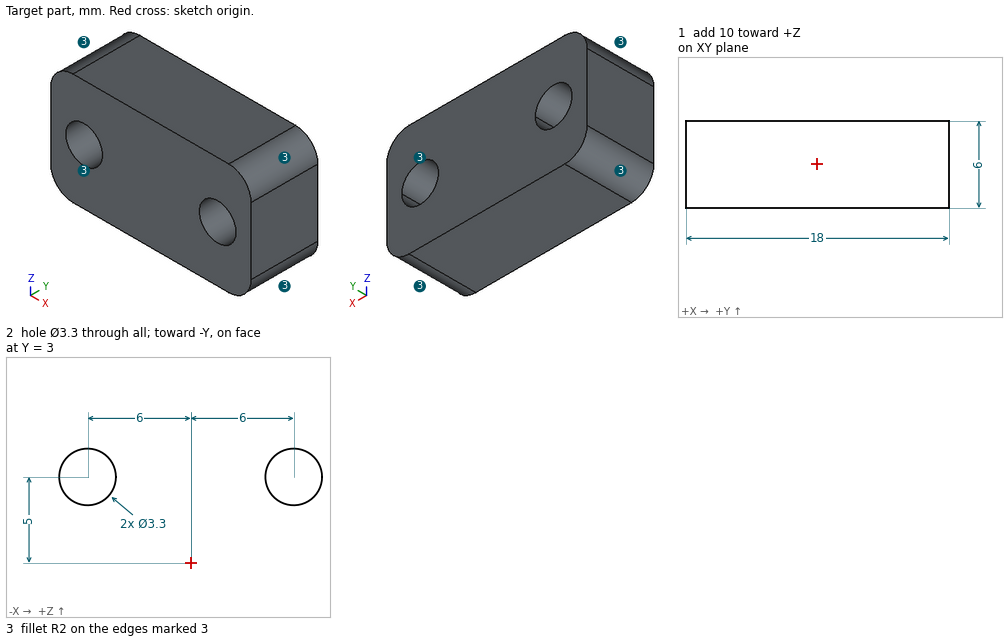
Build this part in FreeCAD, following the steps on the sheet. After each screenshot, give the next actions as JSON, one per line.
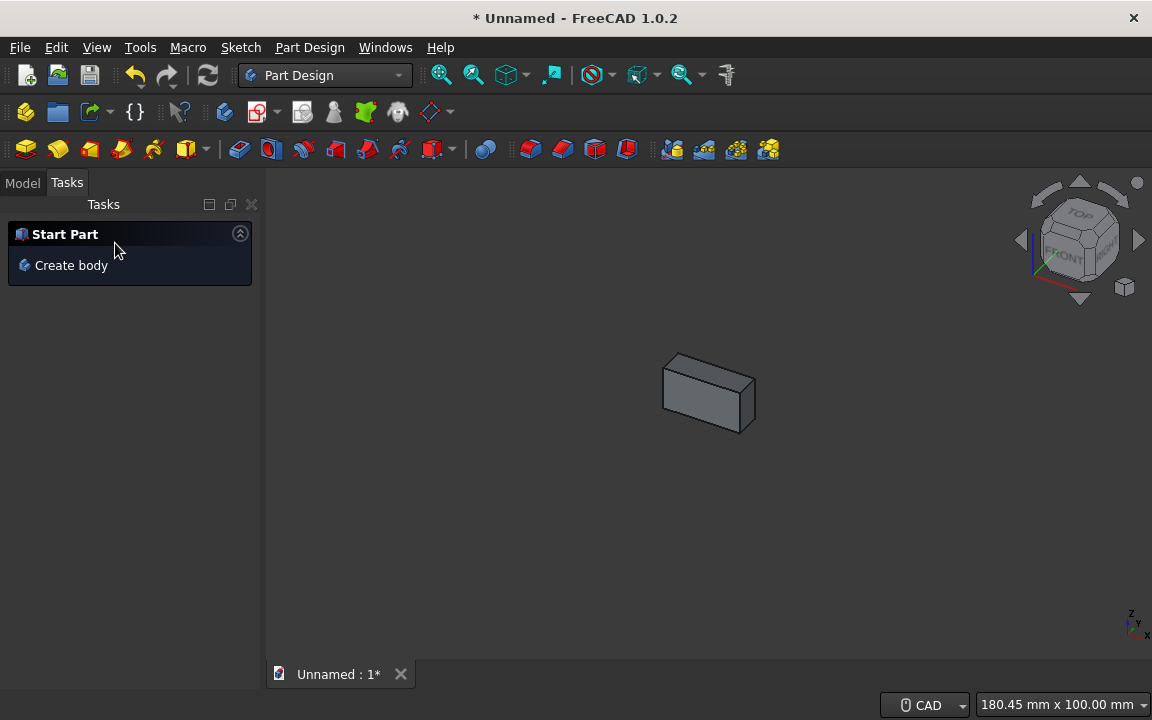
{"action": "key", "text": "v f"}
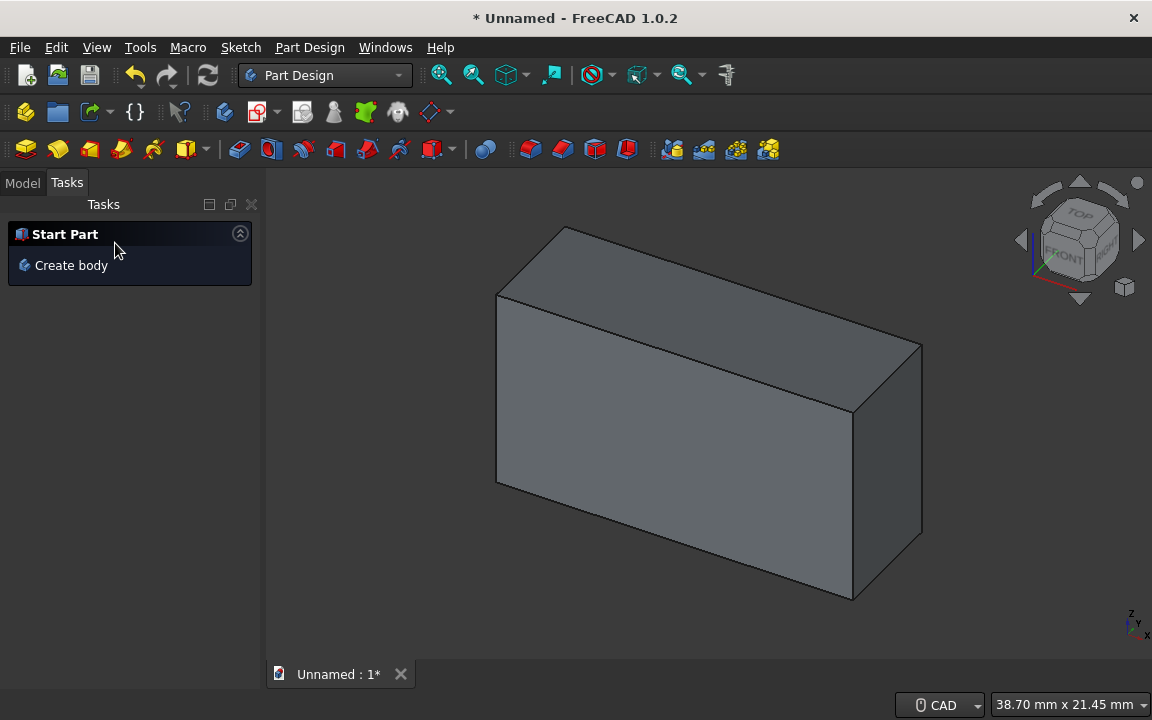
{"action": "key", "text": "4"}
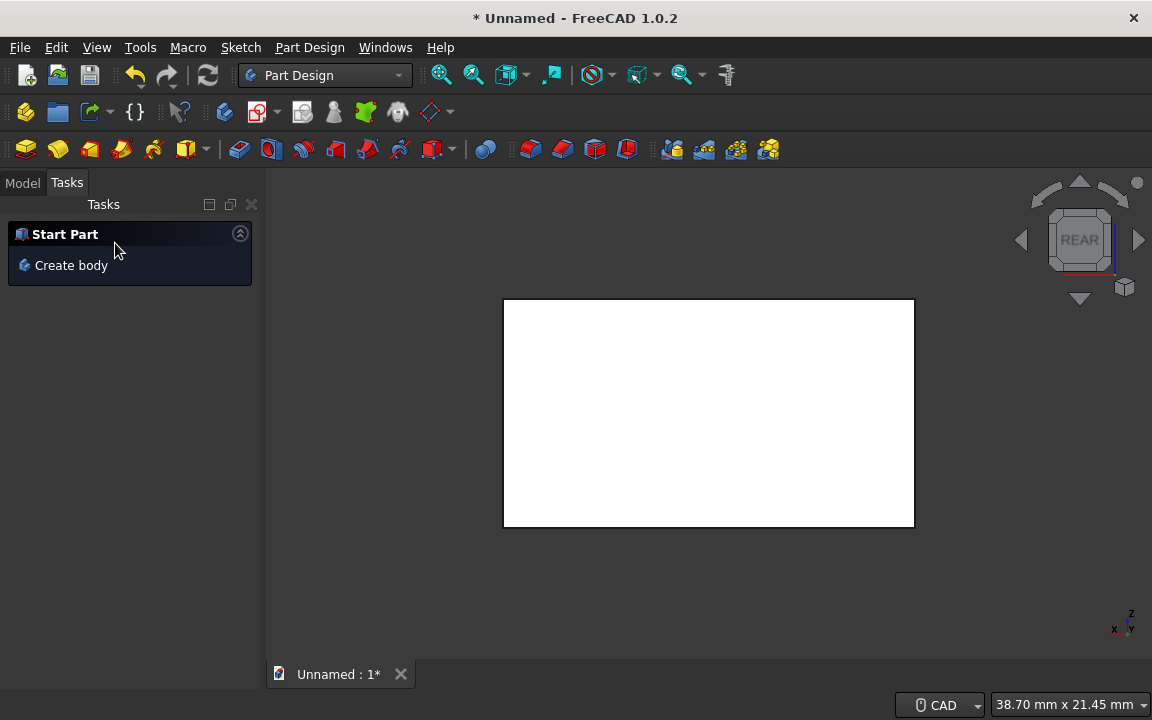
{"action": "left_click", "coordinate": [650, 413]}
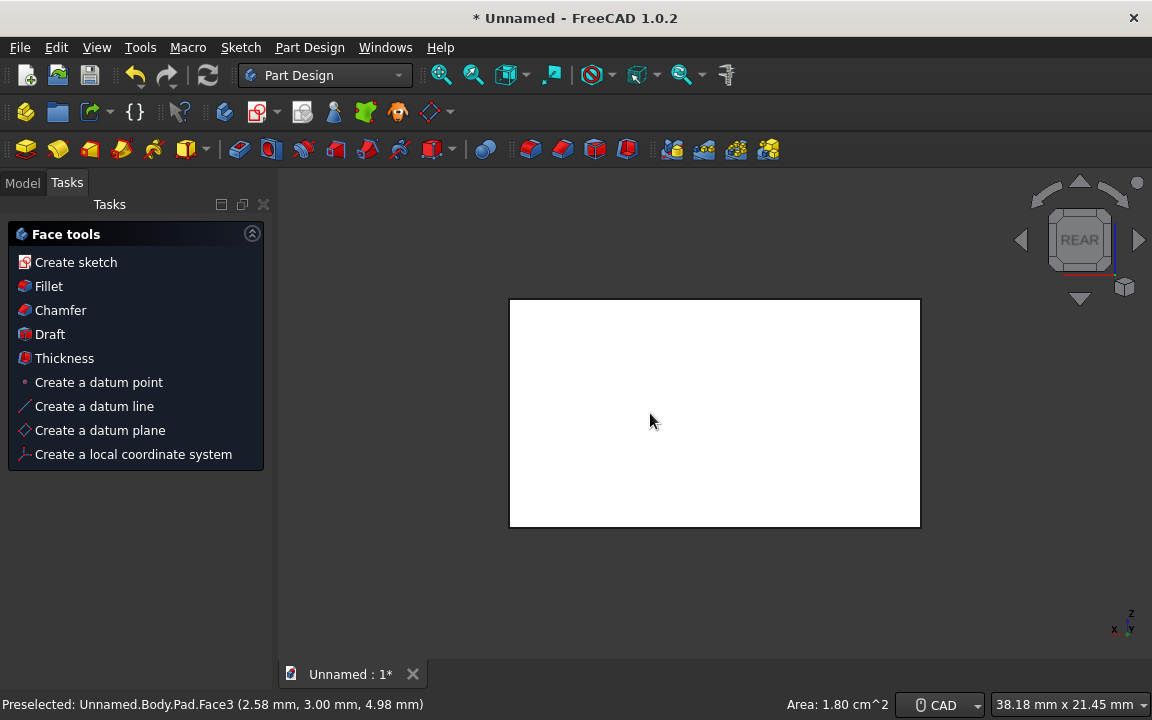
{"action": "left_click", "coordinate": [258, 112]}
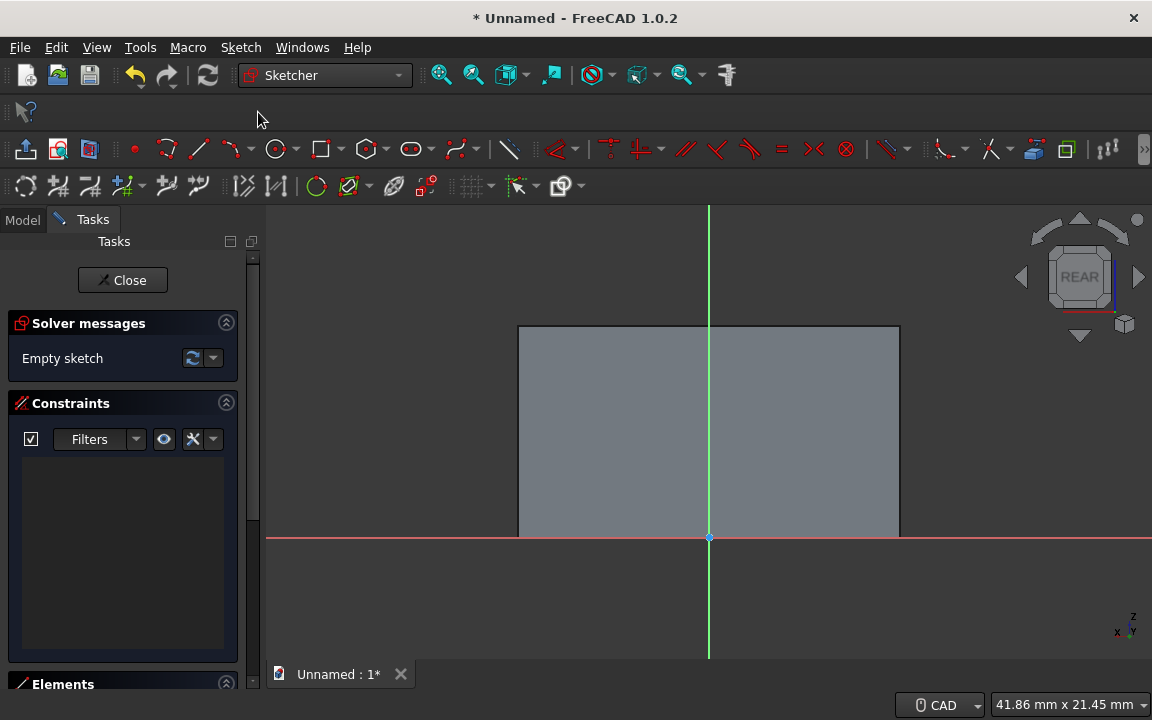
{"action": "scroll", "coordinate": [848, 540], "scroll_direction": "up", "scroll_amount": 2}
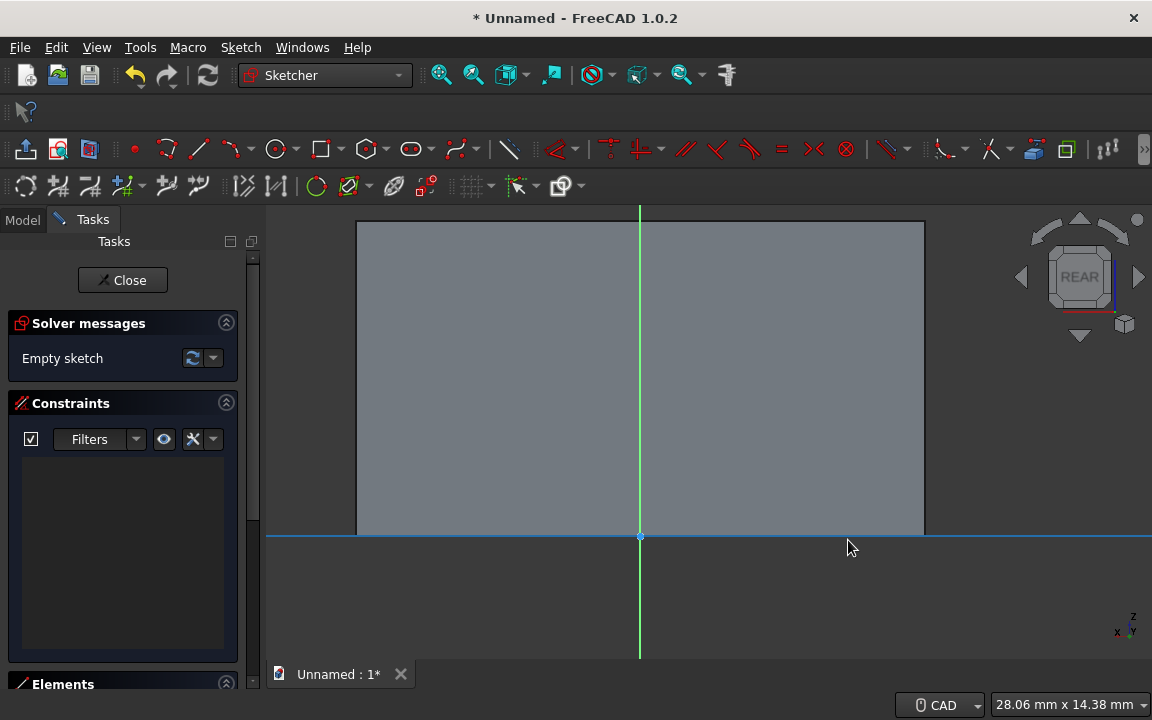
{"action": "left_click", "coordinate": [276, 150]}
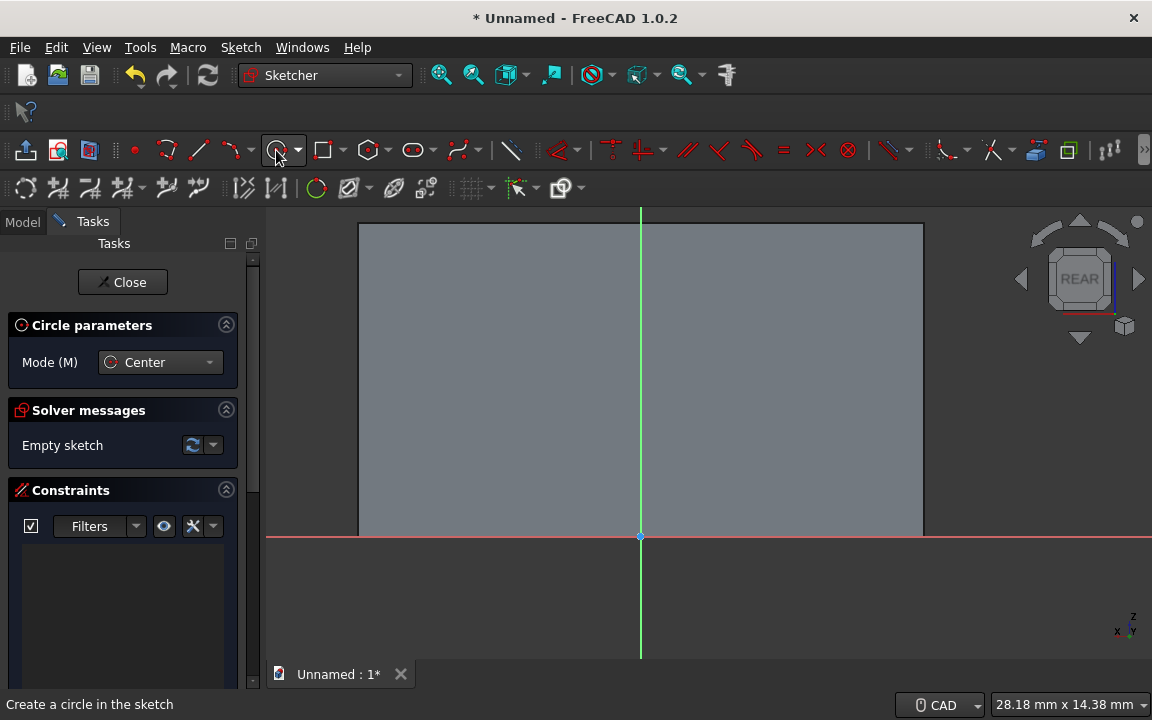
{"action": "left_click", "coordinate": [452, 380]}
{"action": "mouse_move", "coordinate": [489, 343]}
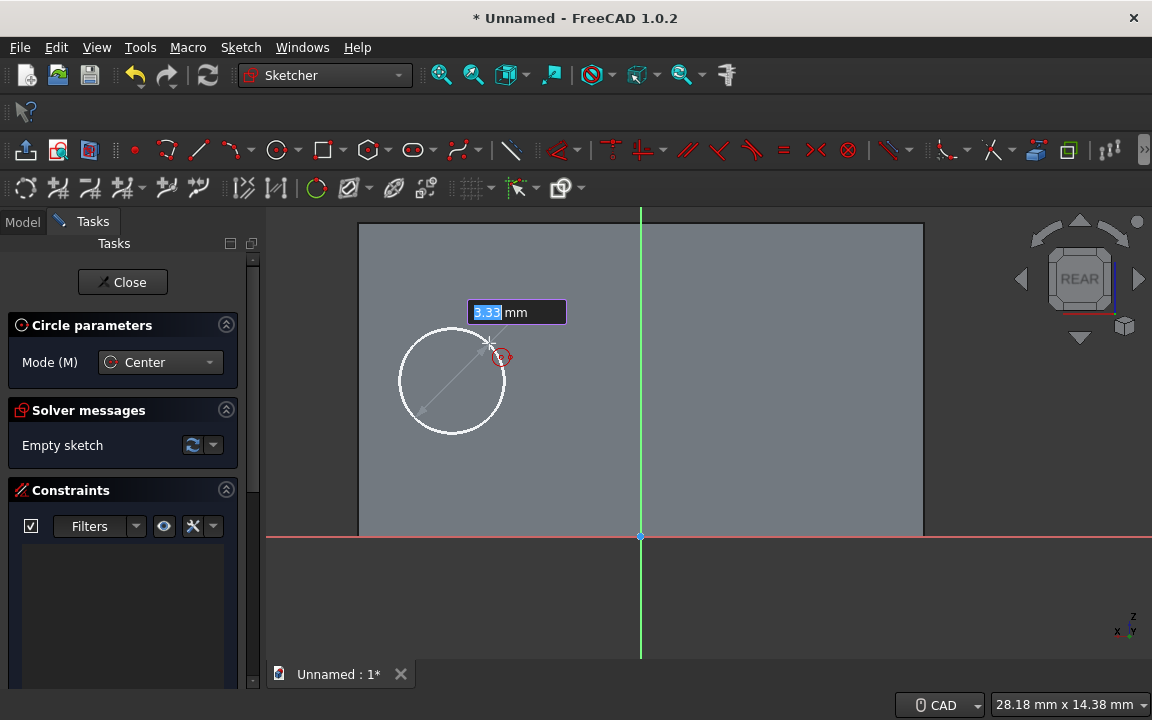
{"action": "type", "text": "3.3"}
{"action": "key", "text": "Return"}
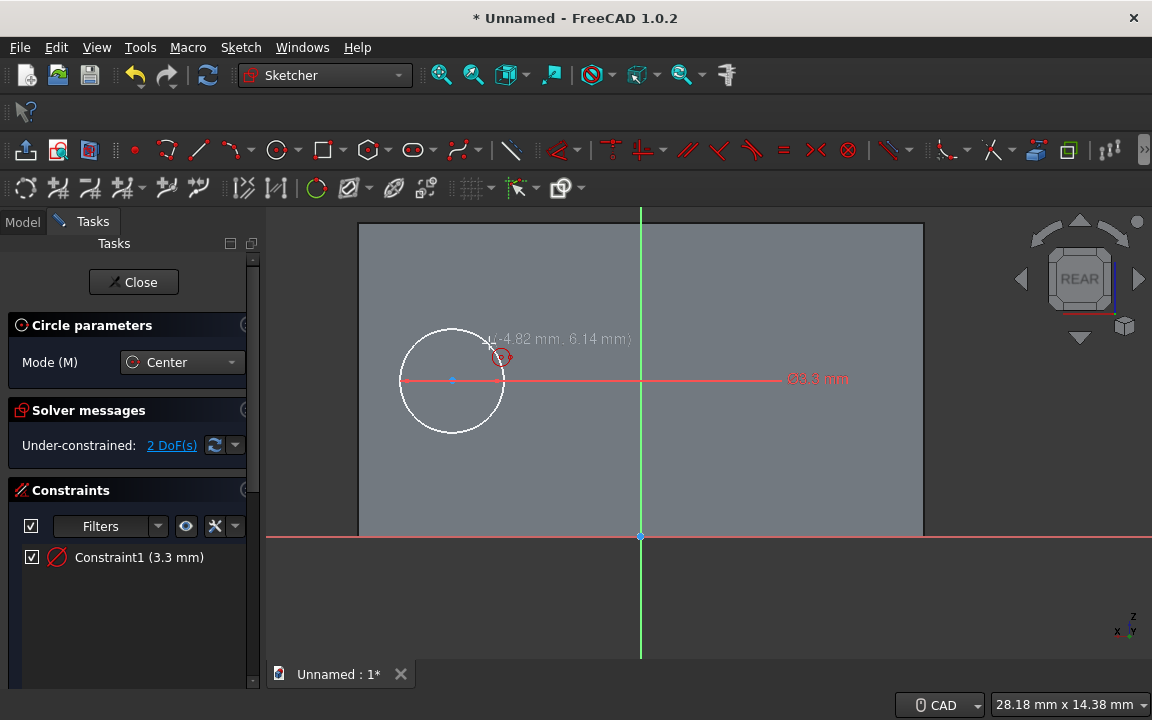
{"action": "left_click", "coordinate": [829, 380]}
{"action": "mouse_move", "coordinate": [866, 343]}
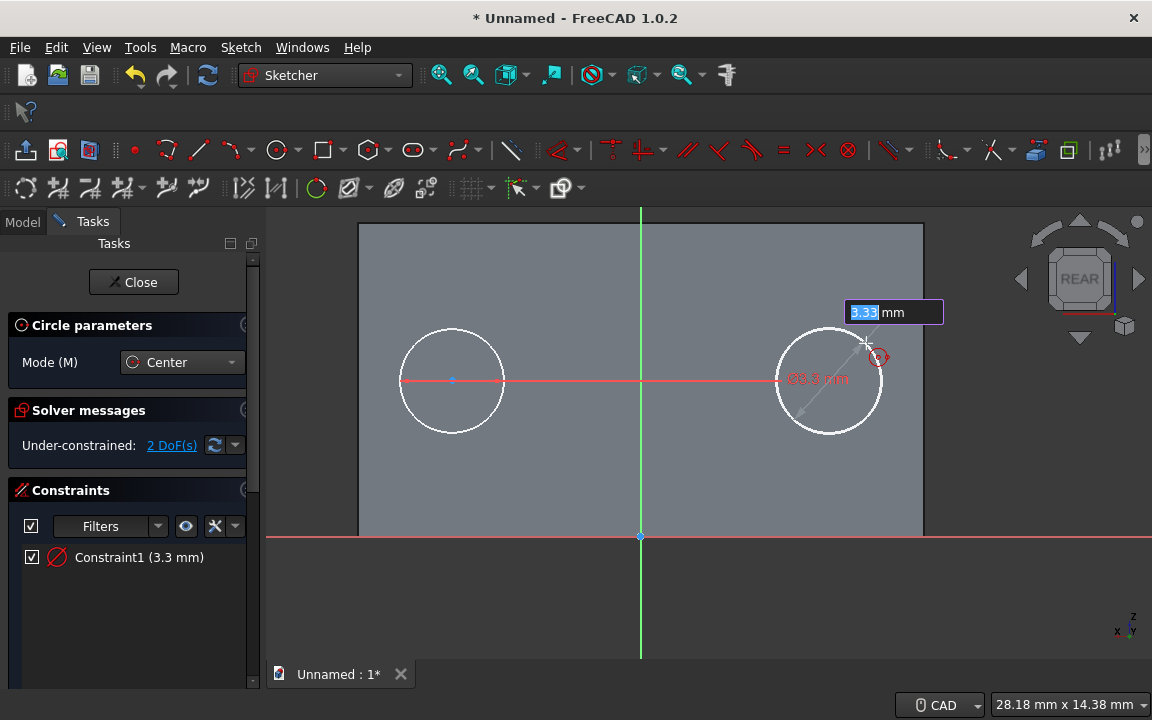
{"action": "type", "text": "3.3"}
{"action": "key", "text": "Return"}
{"action": "key", "text": "Escape"}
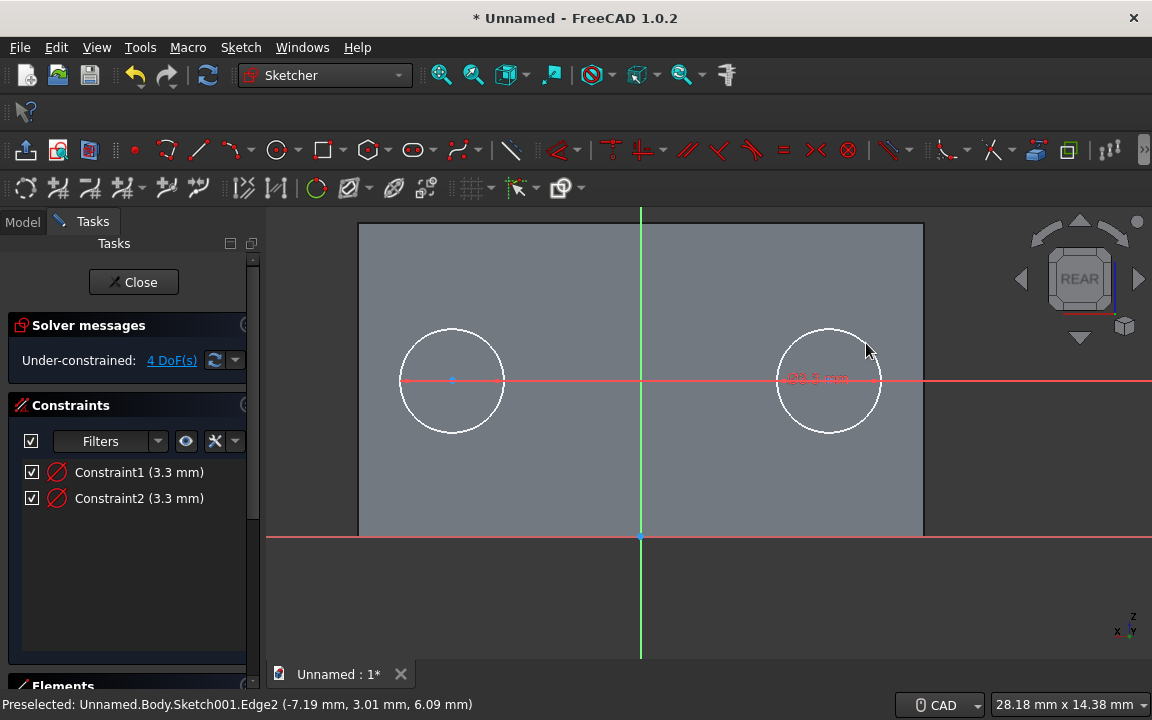
{"action": "left_click", "coordinate": [452, 381]}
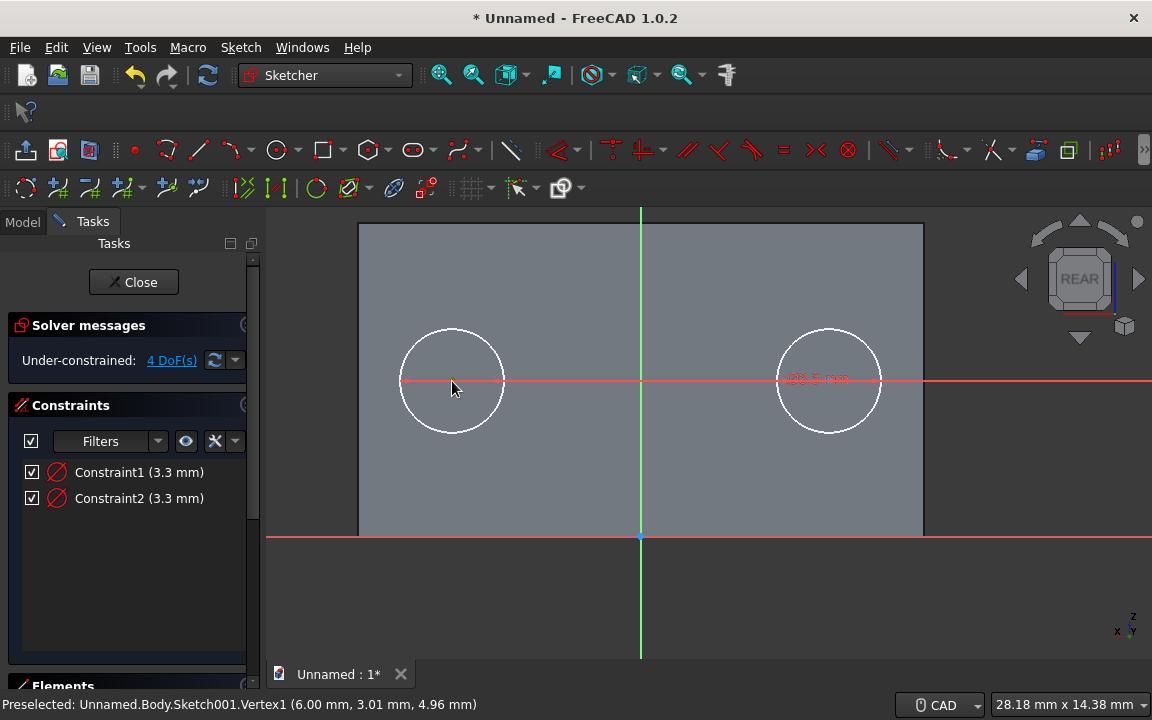
{"action": "left_click", "coordinate": [829, 381]}